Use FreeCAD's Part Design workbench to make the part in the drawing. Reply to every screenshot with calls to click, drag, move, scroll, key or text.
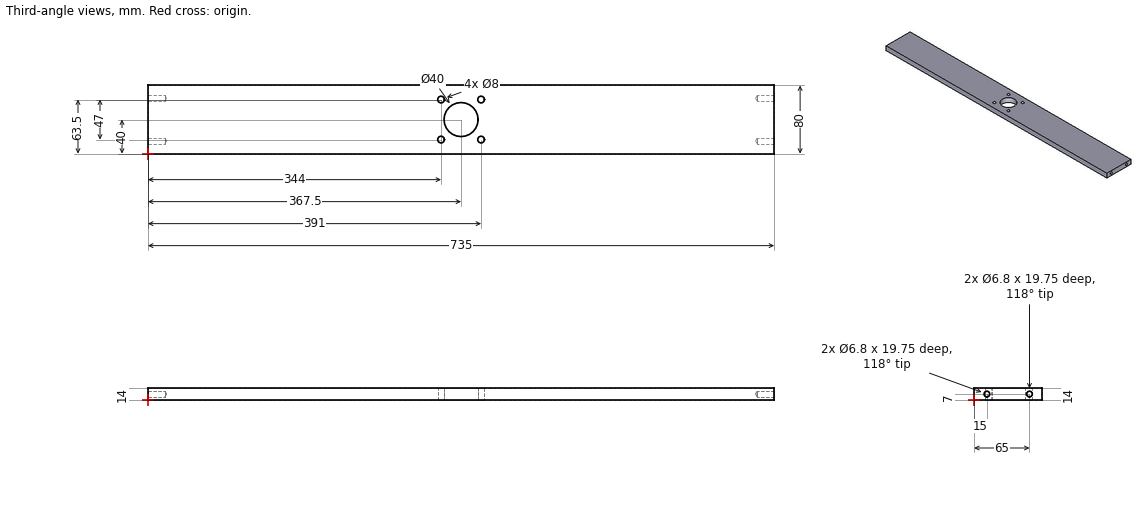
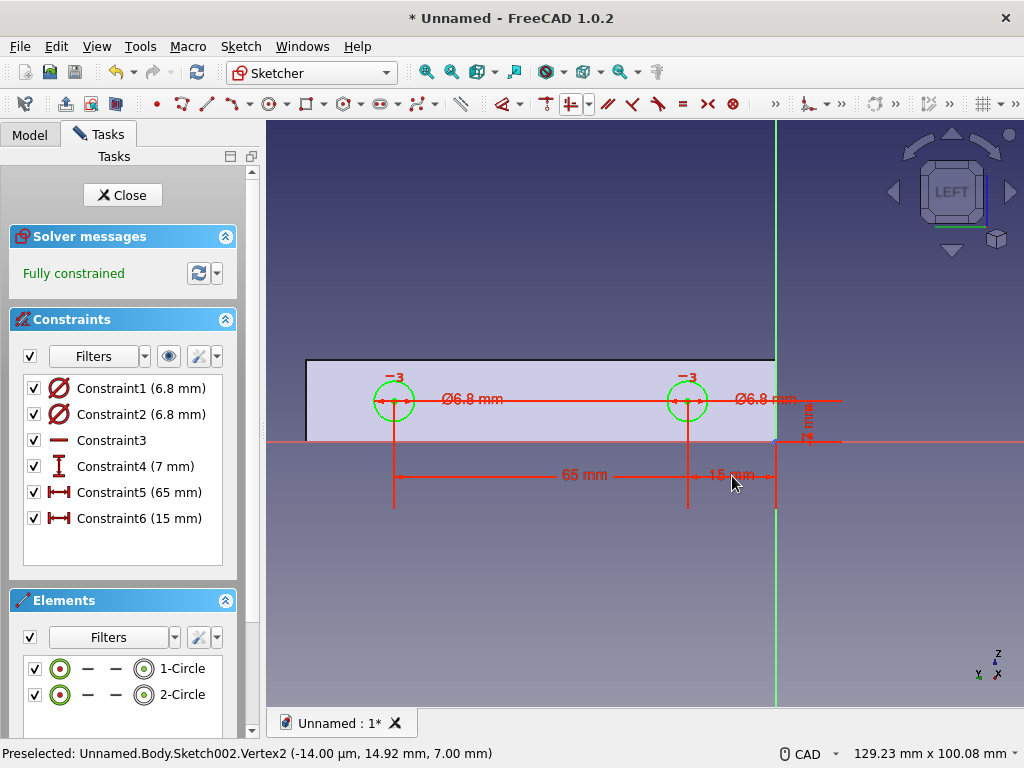
click(123, 195)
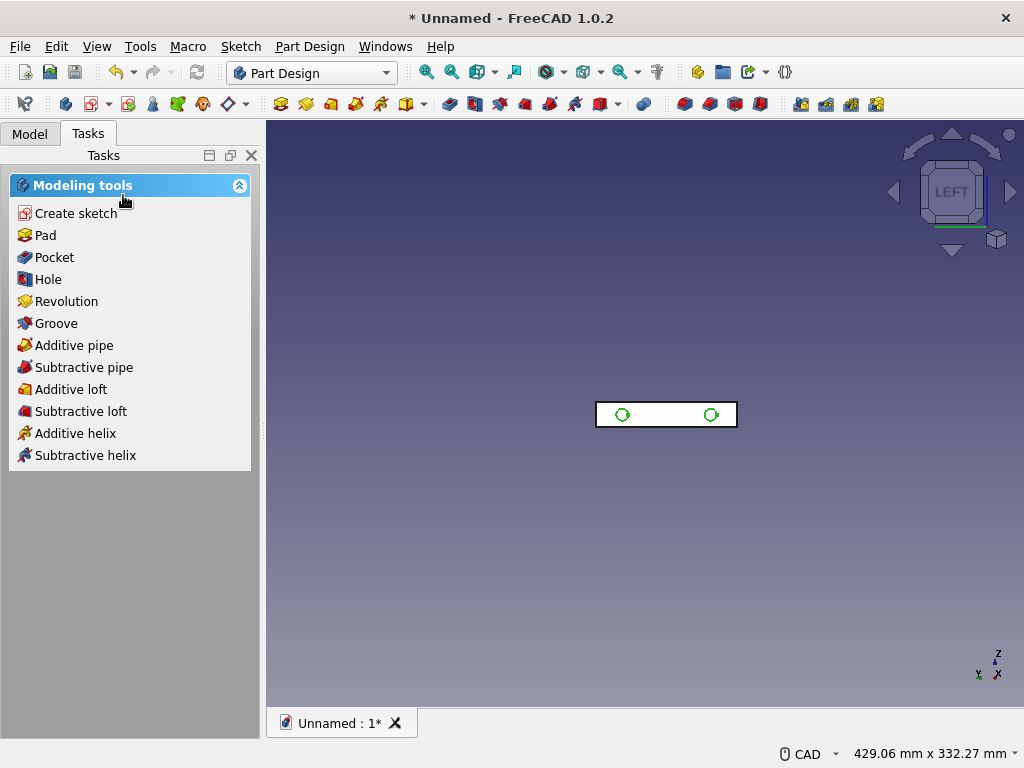
click(475, 104)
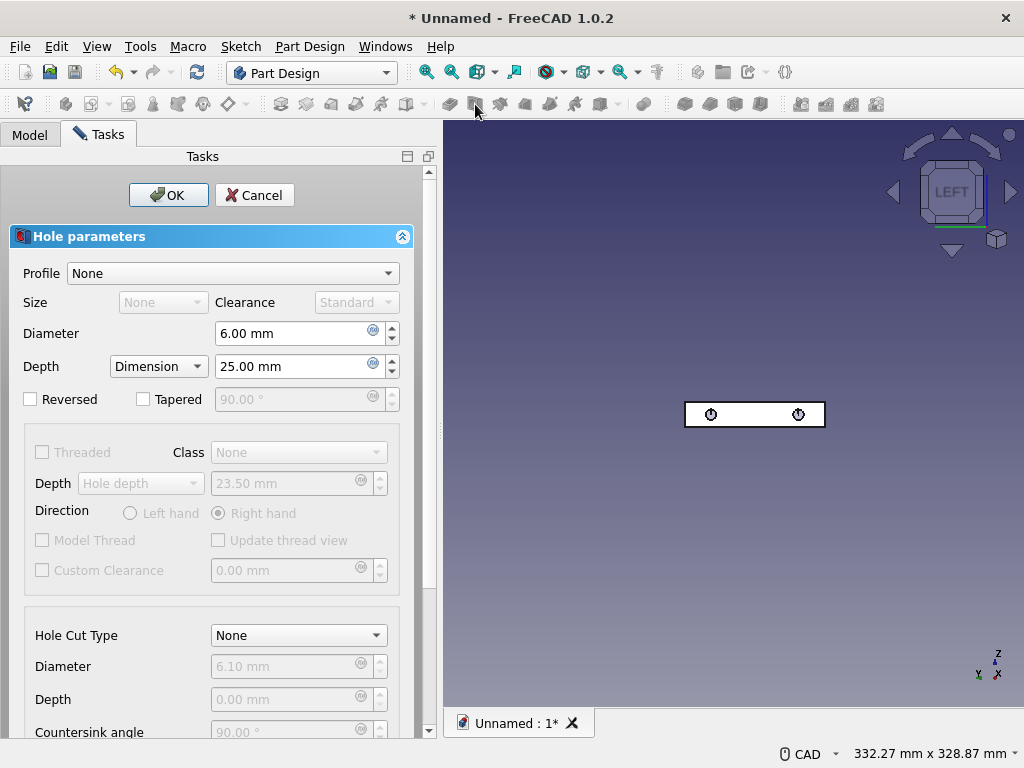
triple_click(300, 334)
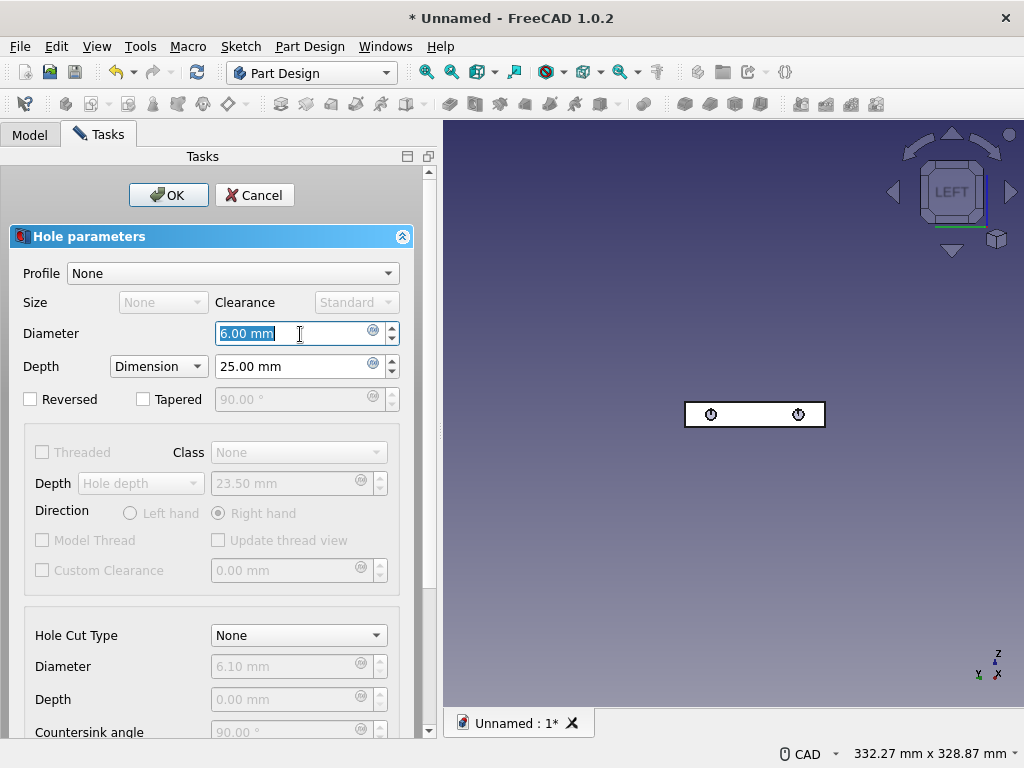
text(6.8)
key(Tab)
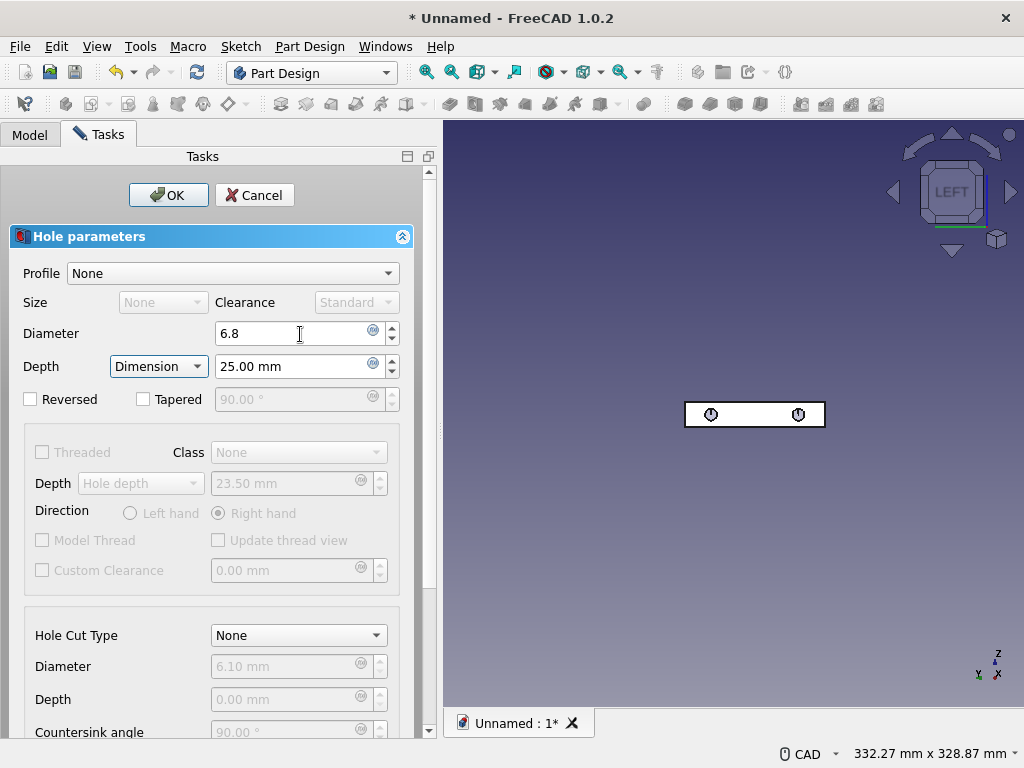
triple_click(300, 366)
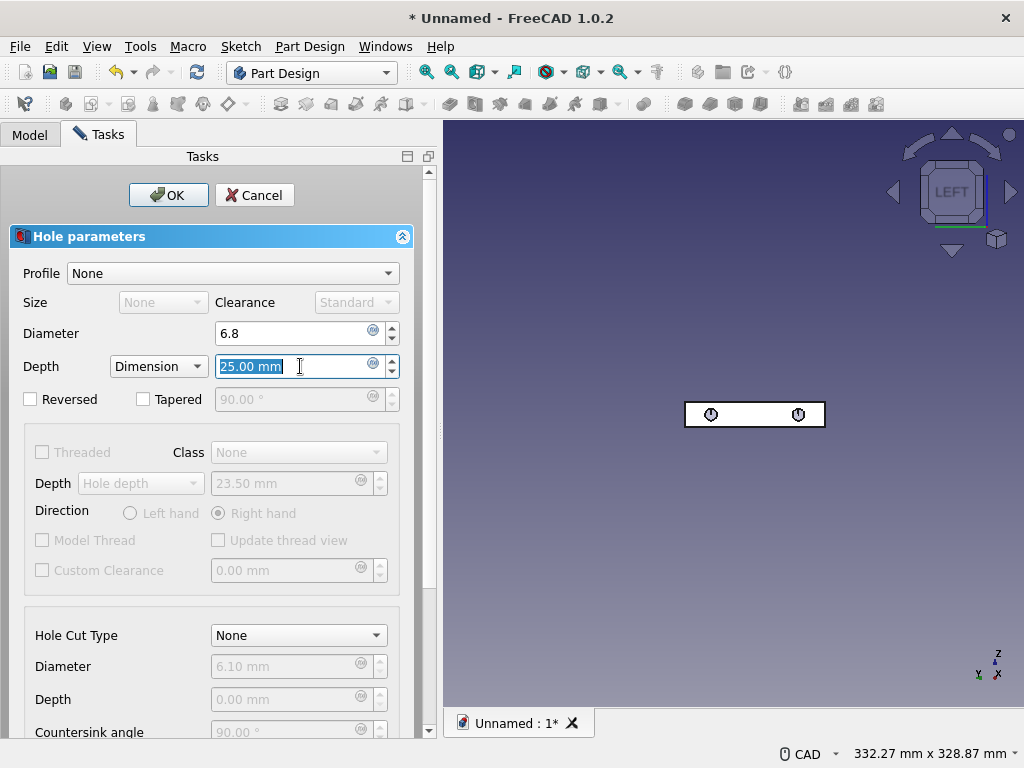
text(19.75)
key(Tab)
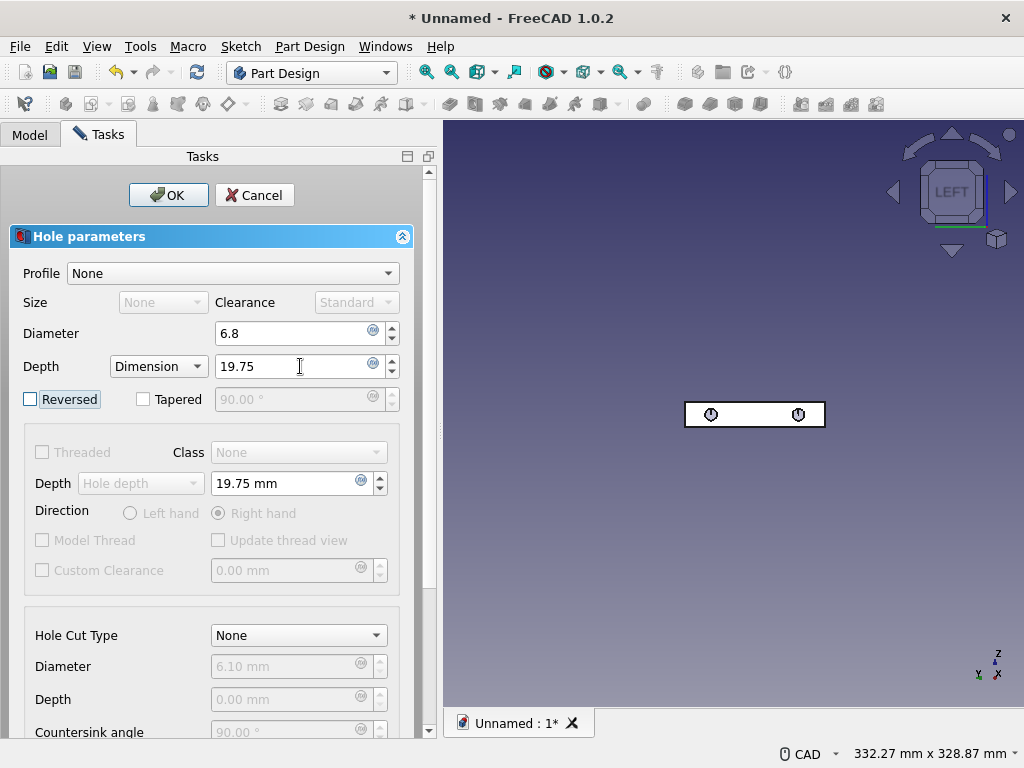
click(169, 195)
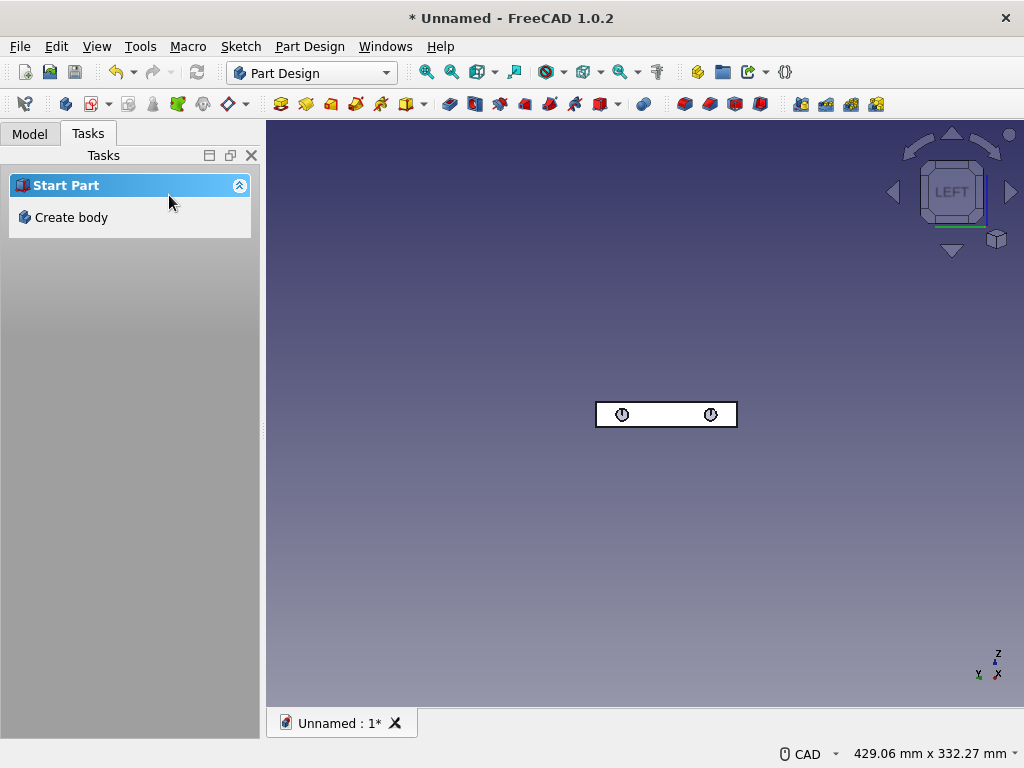
click(427, 72)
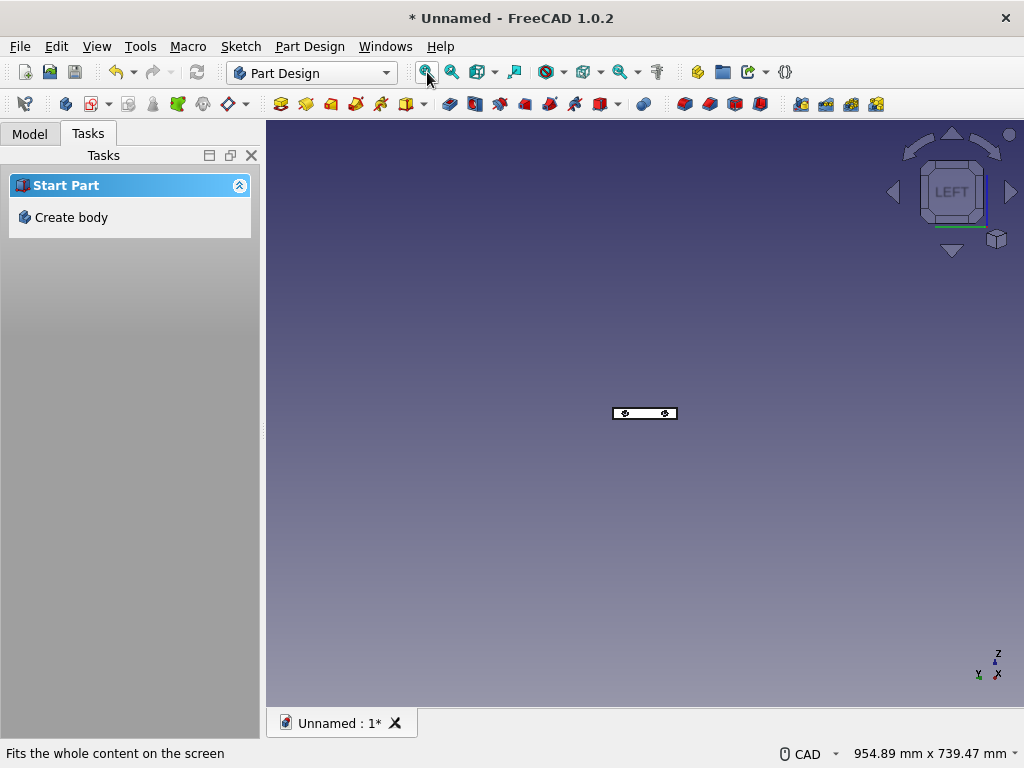
key(0)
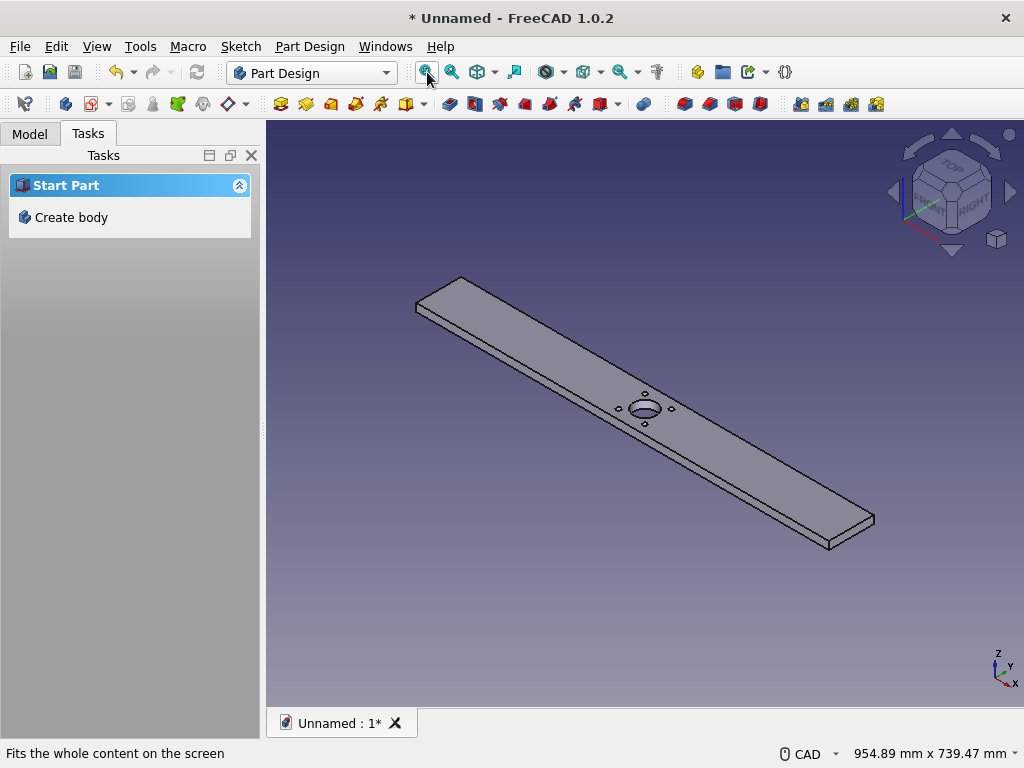
key(3)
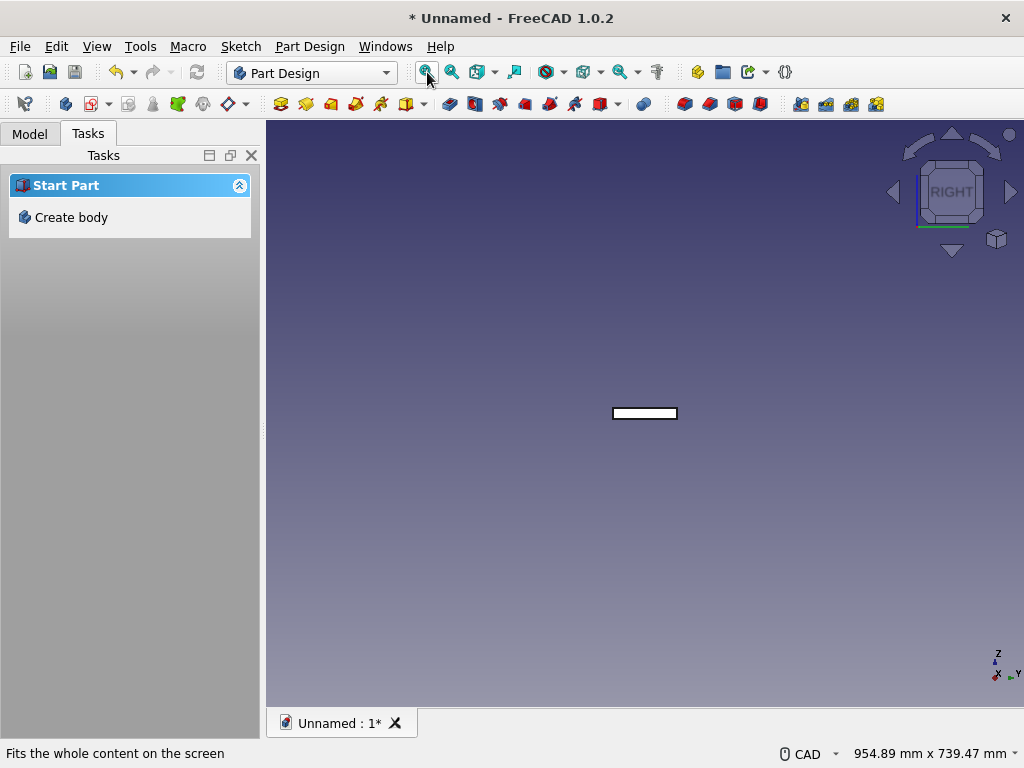
click(427, 72)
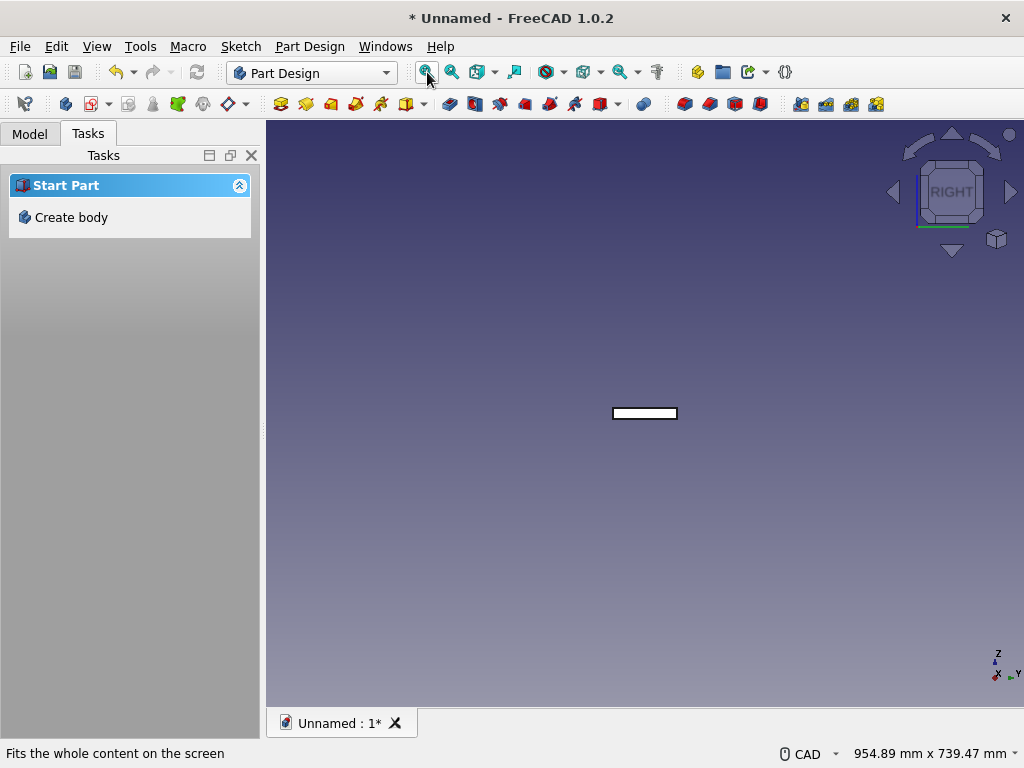
scroll(663, 412, up, 4)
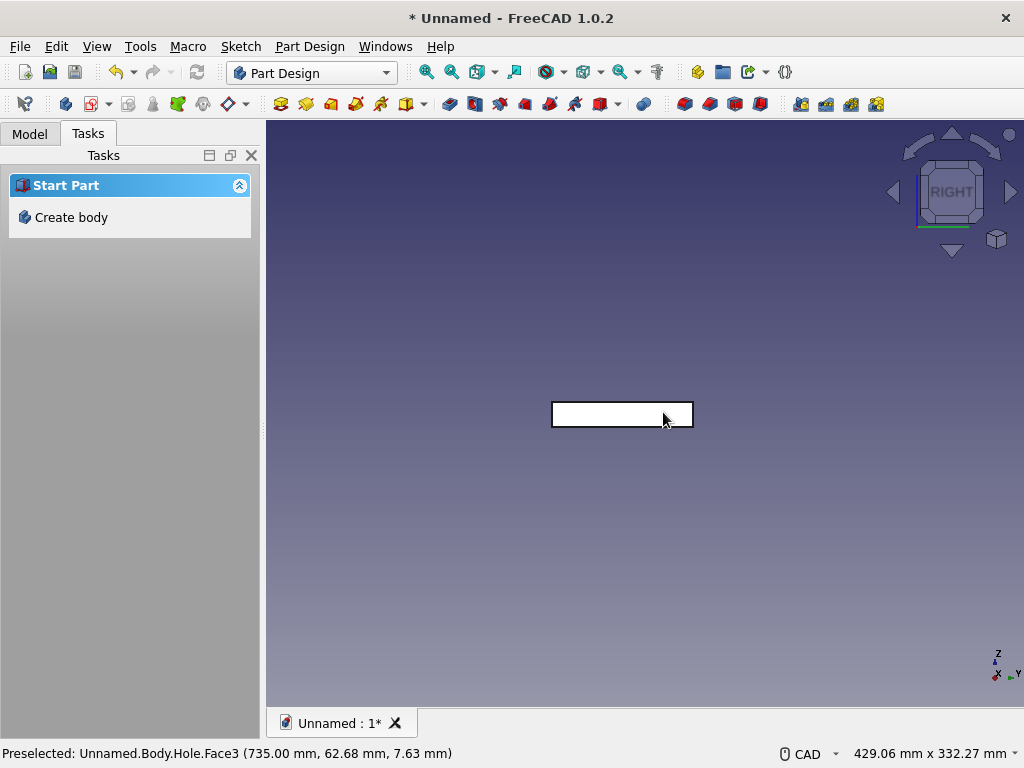
click(663, 414)